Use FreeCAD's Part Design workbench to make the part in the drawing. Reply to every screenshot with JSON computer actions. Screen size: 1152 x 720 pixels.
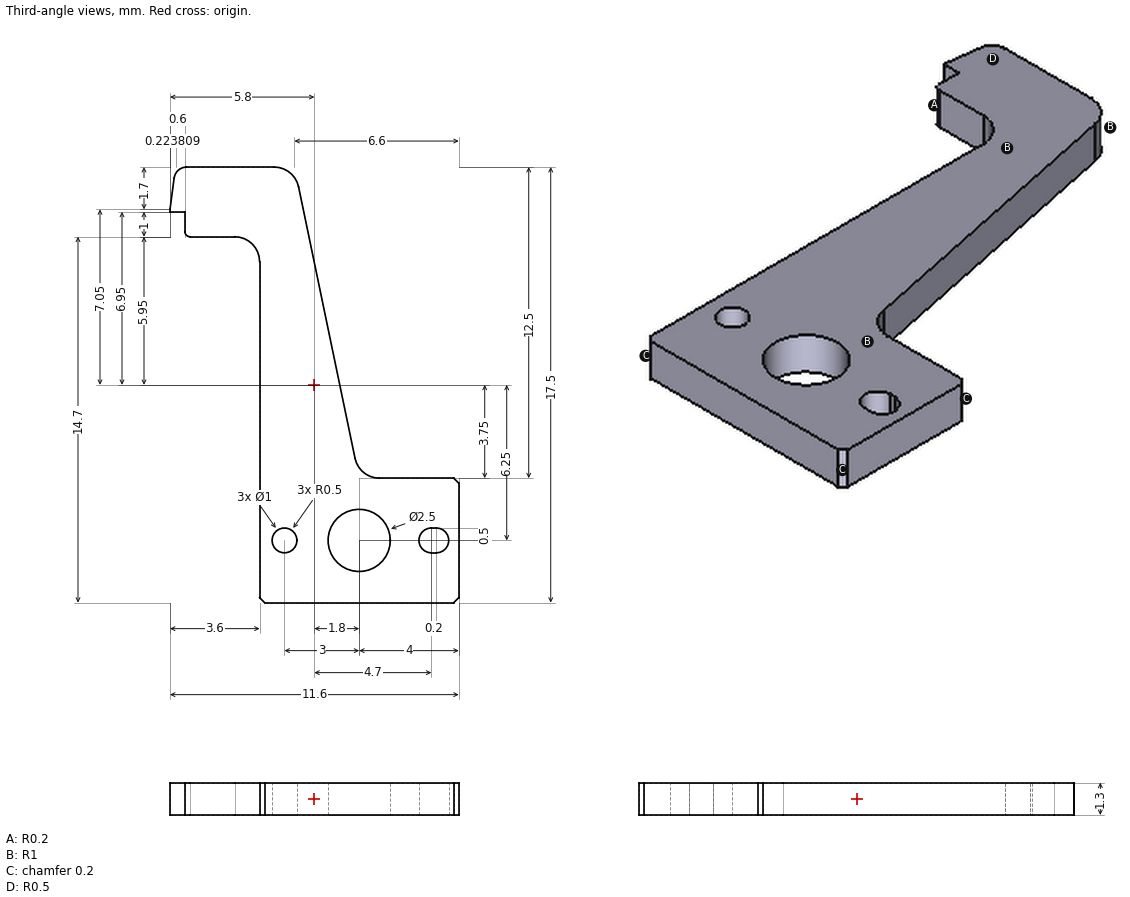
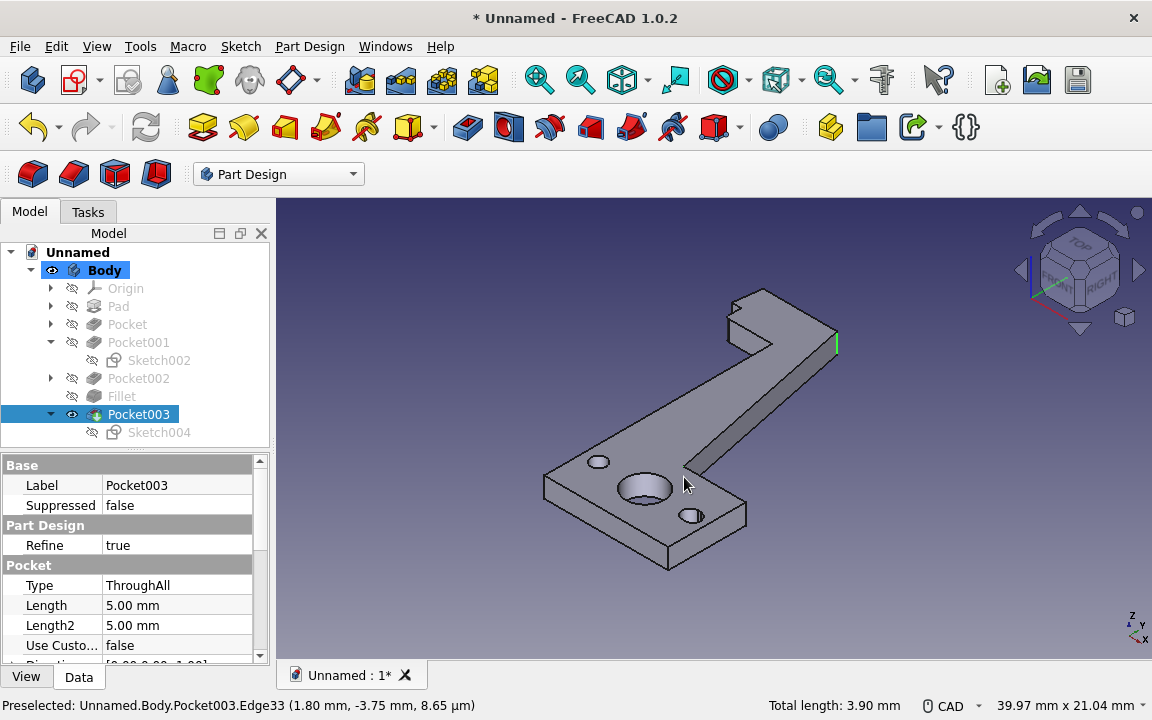
{"action": "left_click", "coordinate": [33, 174]}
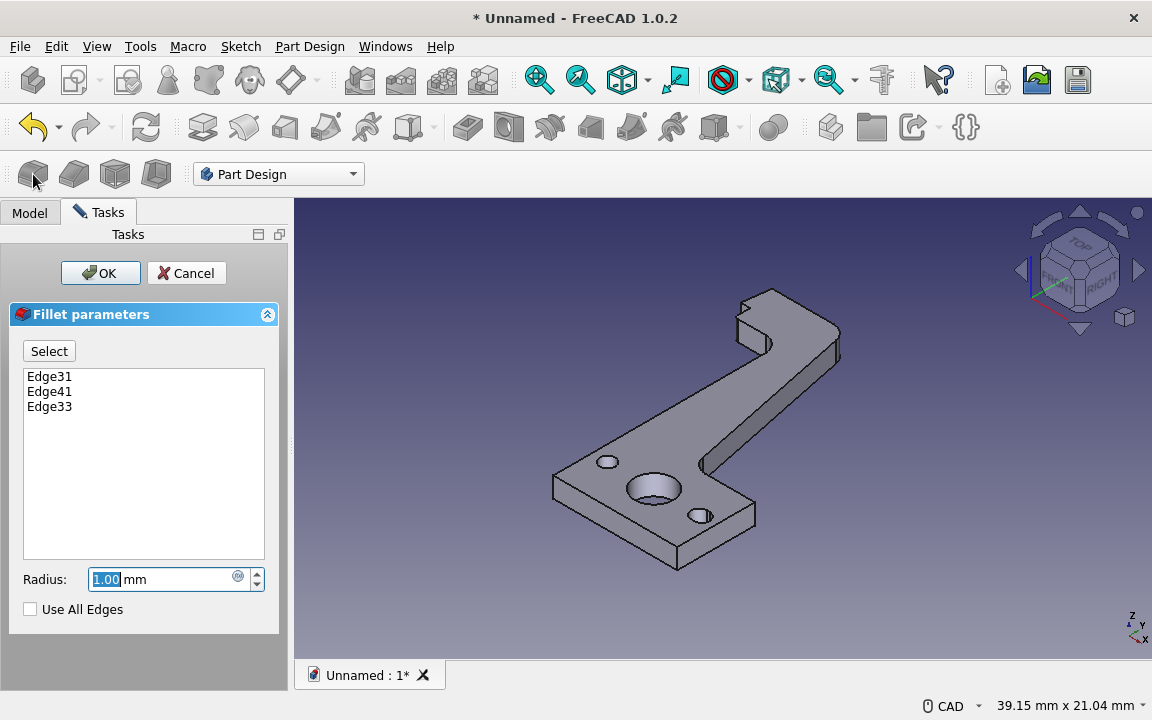
{"action": "type", "text": "1"}
{"action": "key", "text": "Tab"}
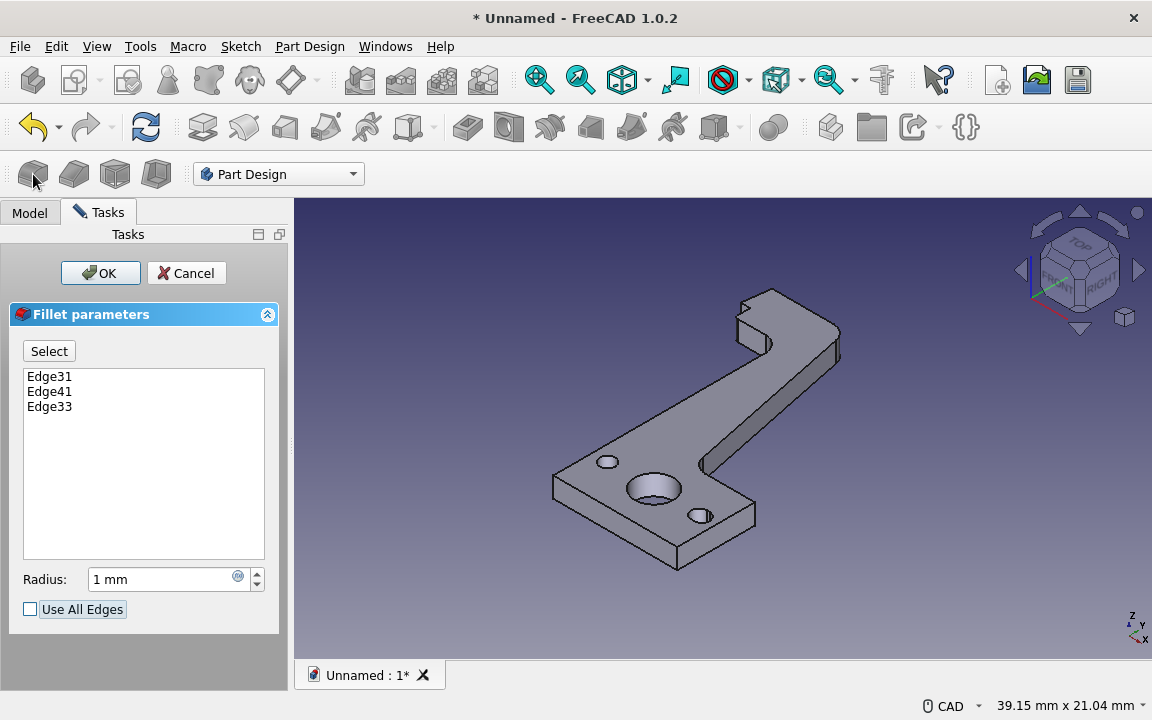
{"action": "left_click", "coordinate": [101, 273]}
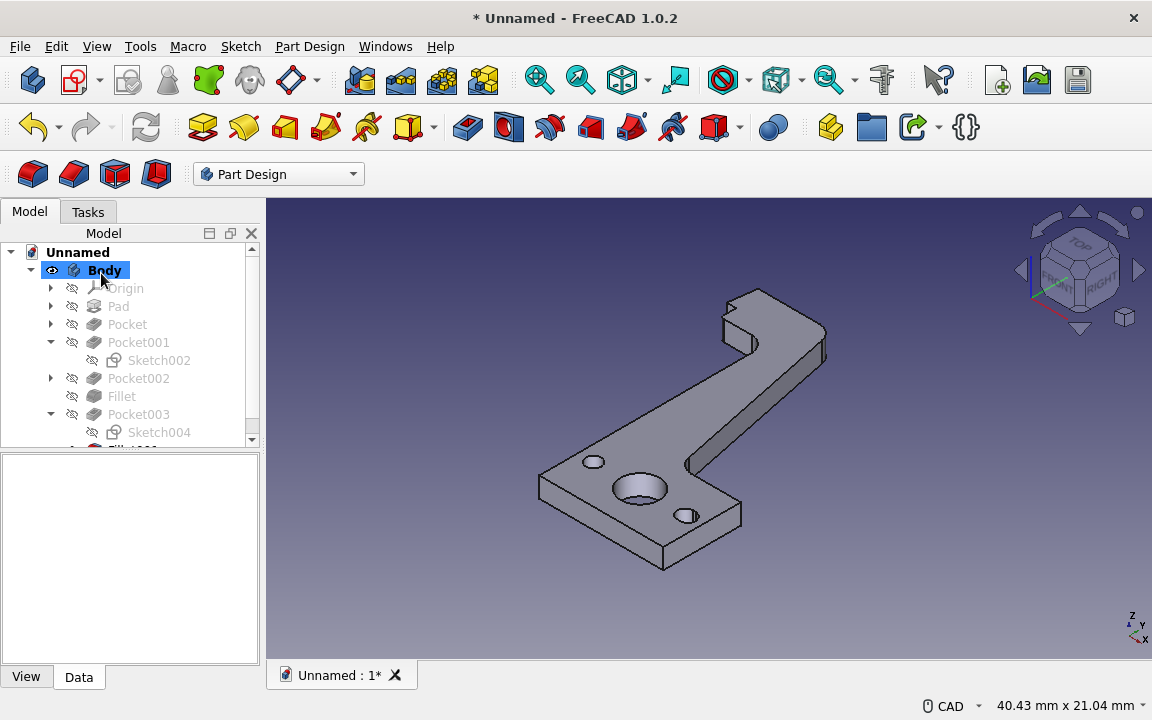
{"action": "left_click", "coordinate": [663, 558]}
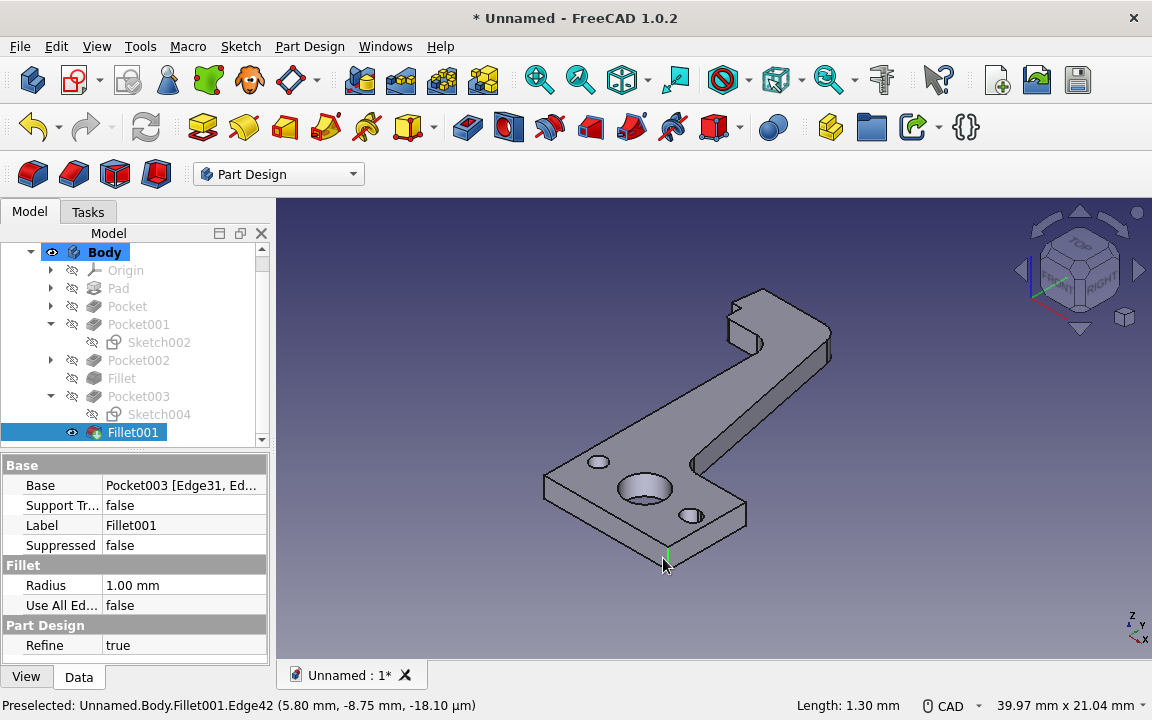
{"action": "key", "text": "2"}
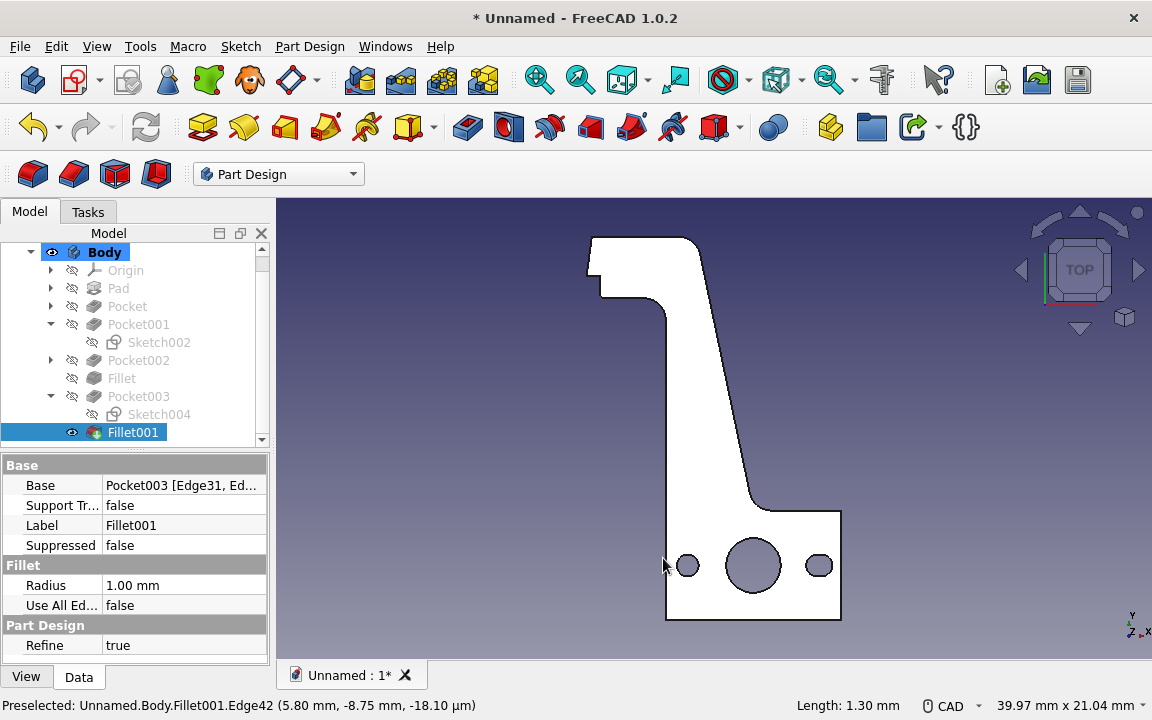
{"action": "key", "text": "0"}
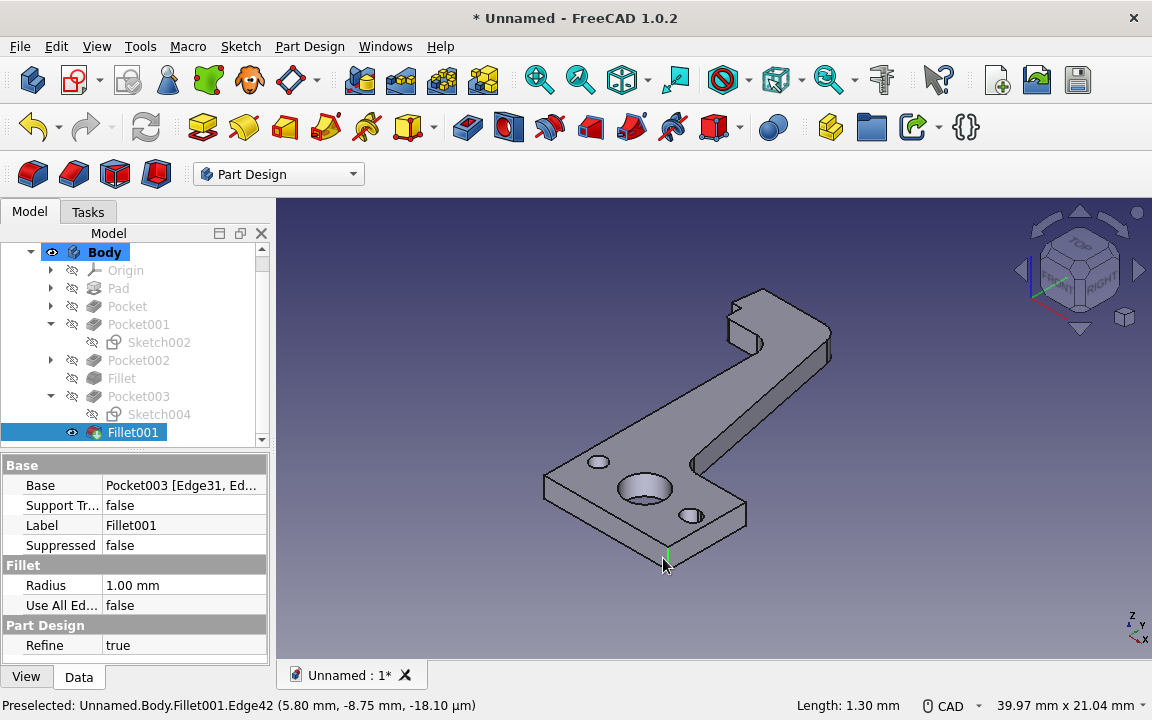
{"action": "key", "text": "1"}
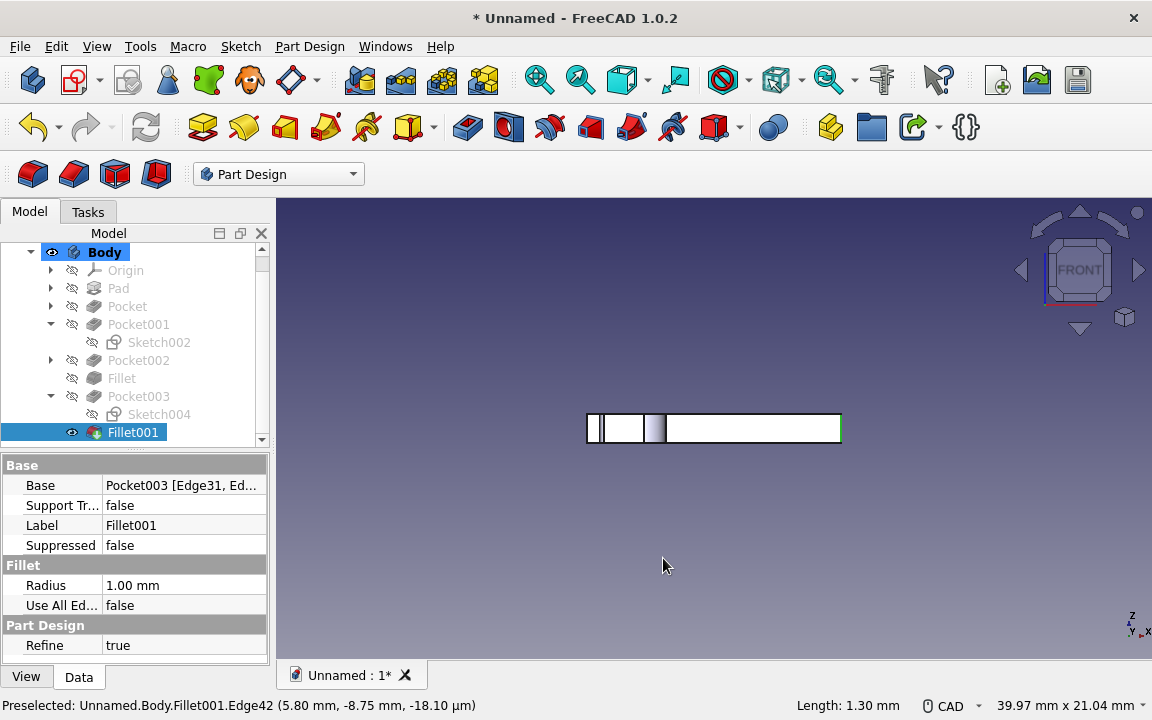
{"action": "key", "text": "v f"}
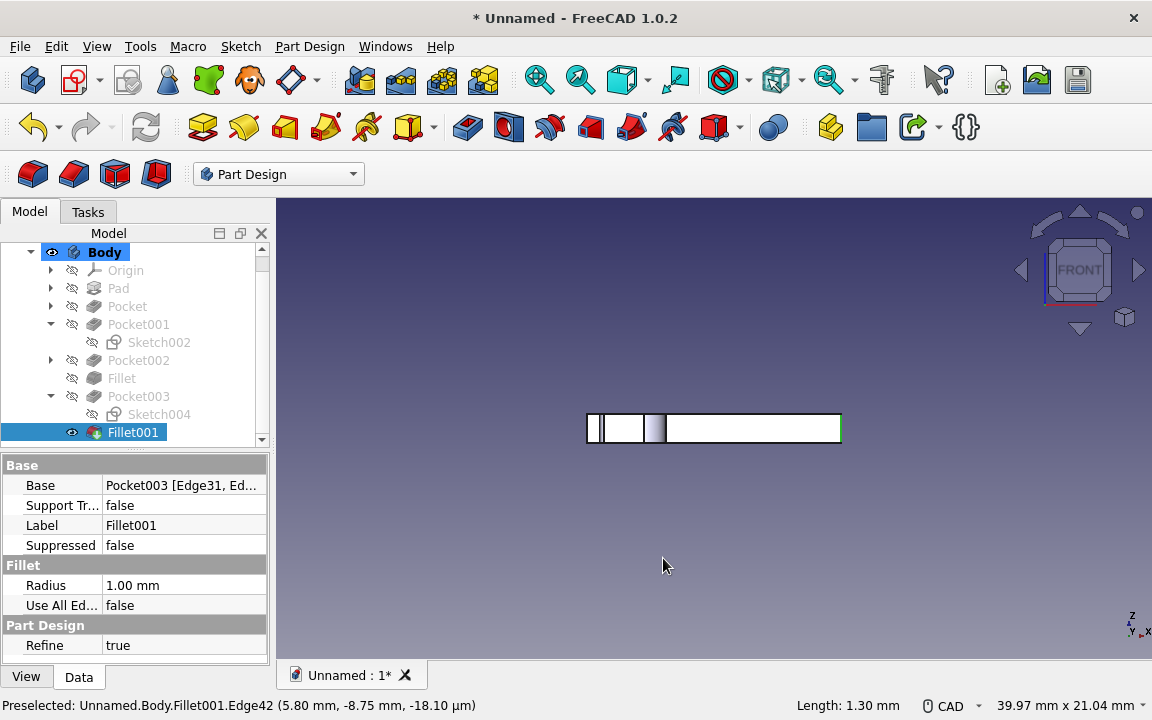
{"action": "left_click", "coordinate": [666, 428], "text": "ctrl"}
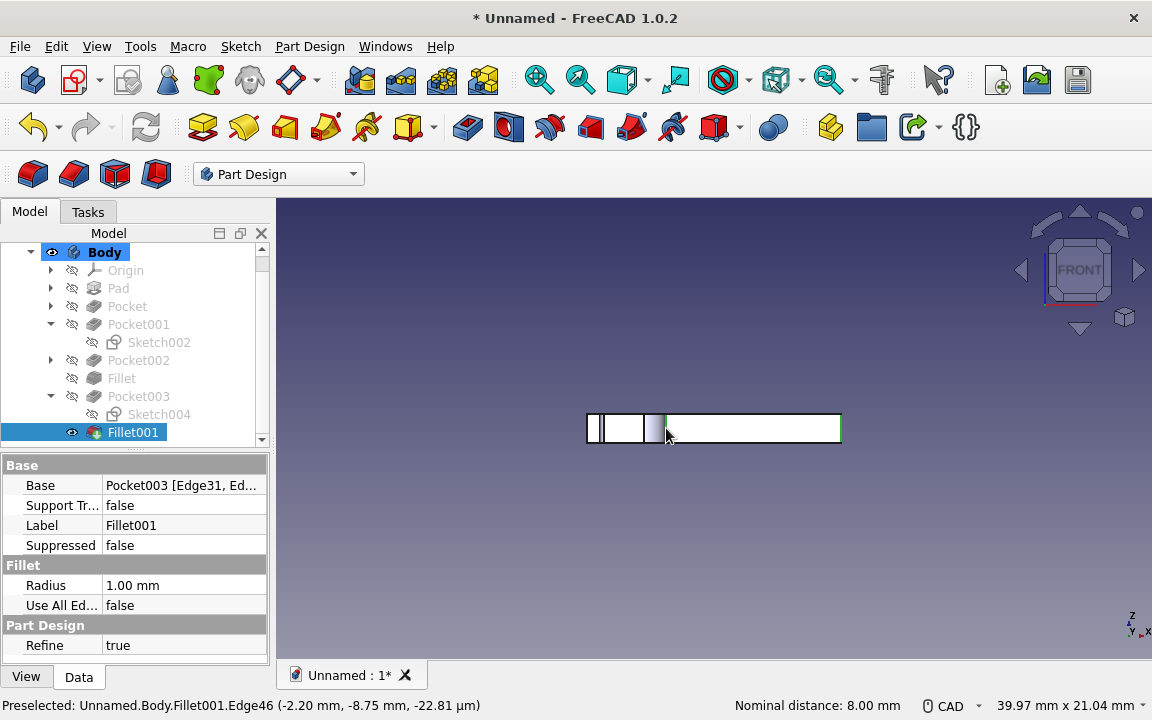
{"action": "key", "text": "3"}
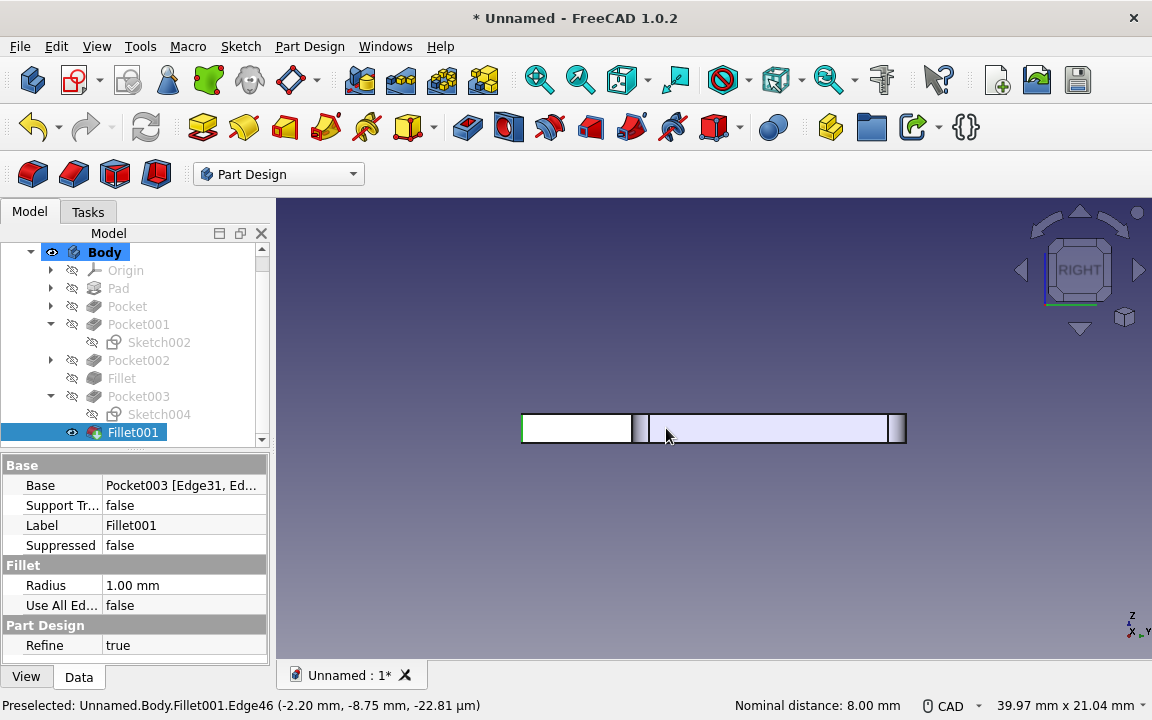
{"action": "left_click", "coordinate": [540, 80]}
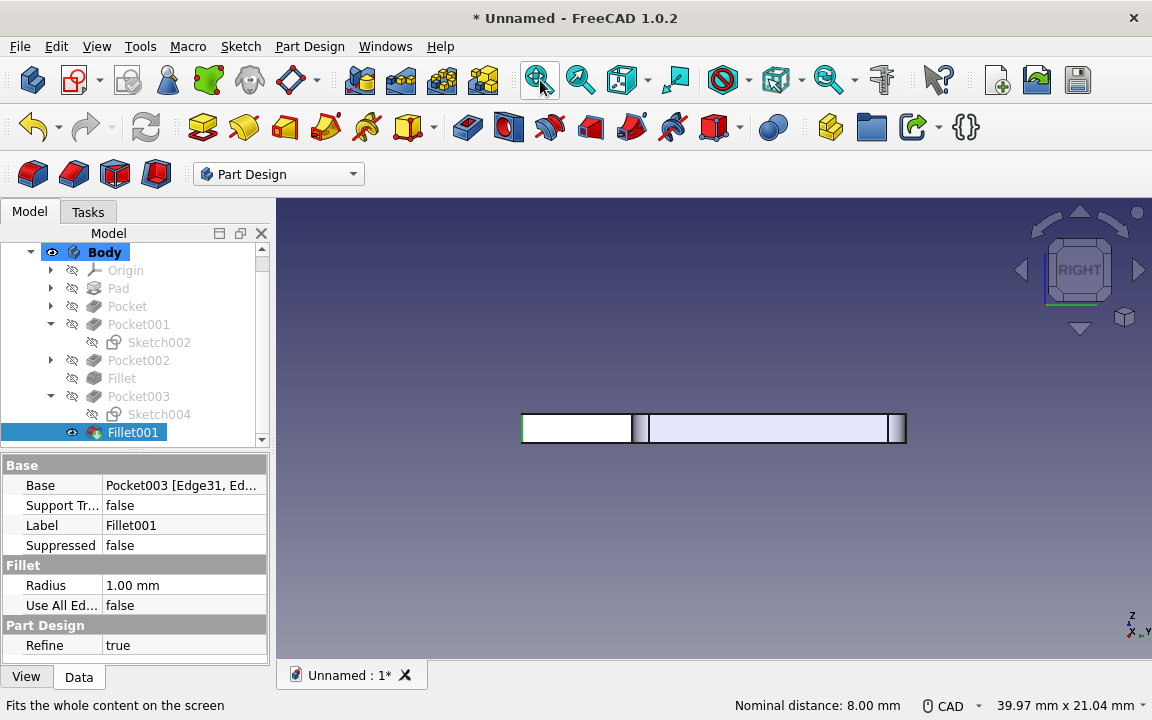
{"action": "left_click", "coordinate": [632, 427], "text": "ctrl"}